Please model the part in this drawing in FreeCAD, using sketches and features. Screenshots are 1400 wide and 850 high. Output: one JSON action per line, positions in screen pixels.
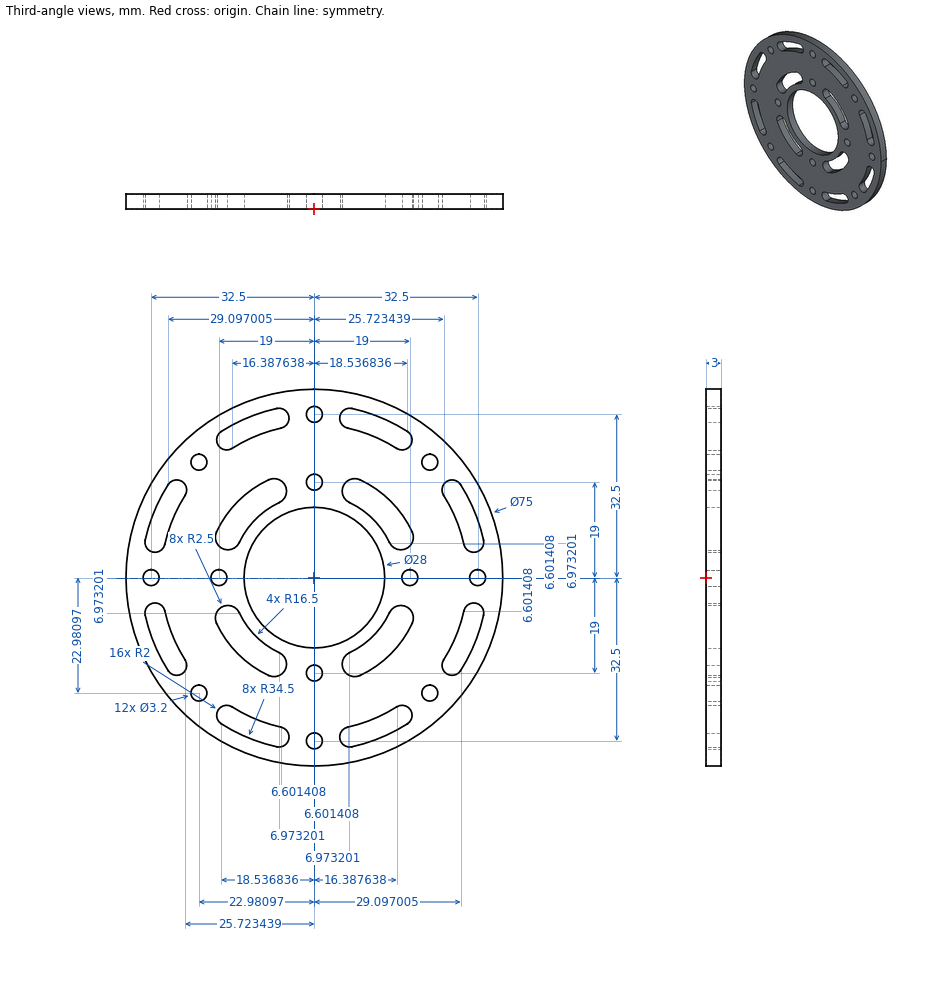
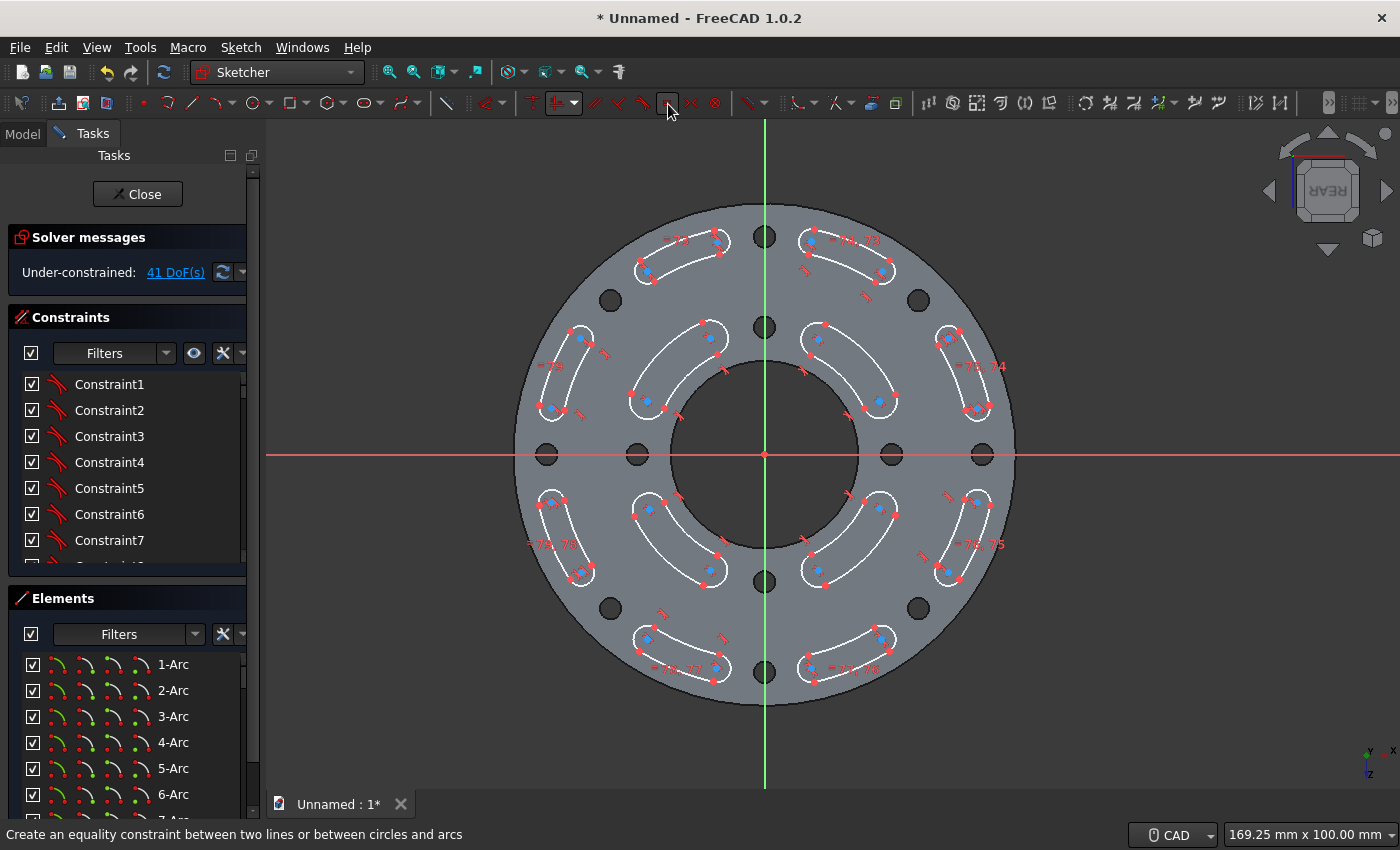
{"action": "scroll", "coordinate": [729, 247], "scroll_direction": "up", "scroll_amount": 2}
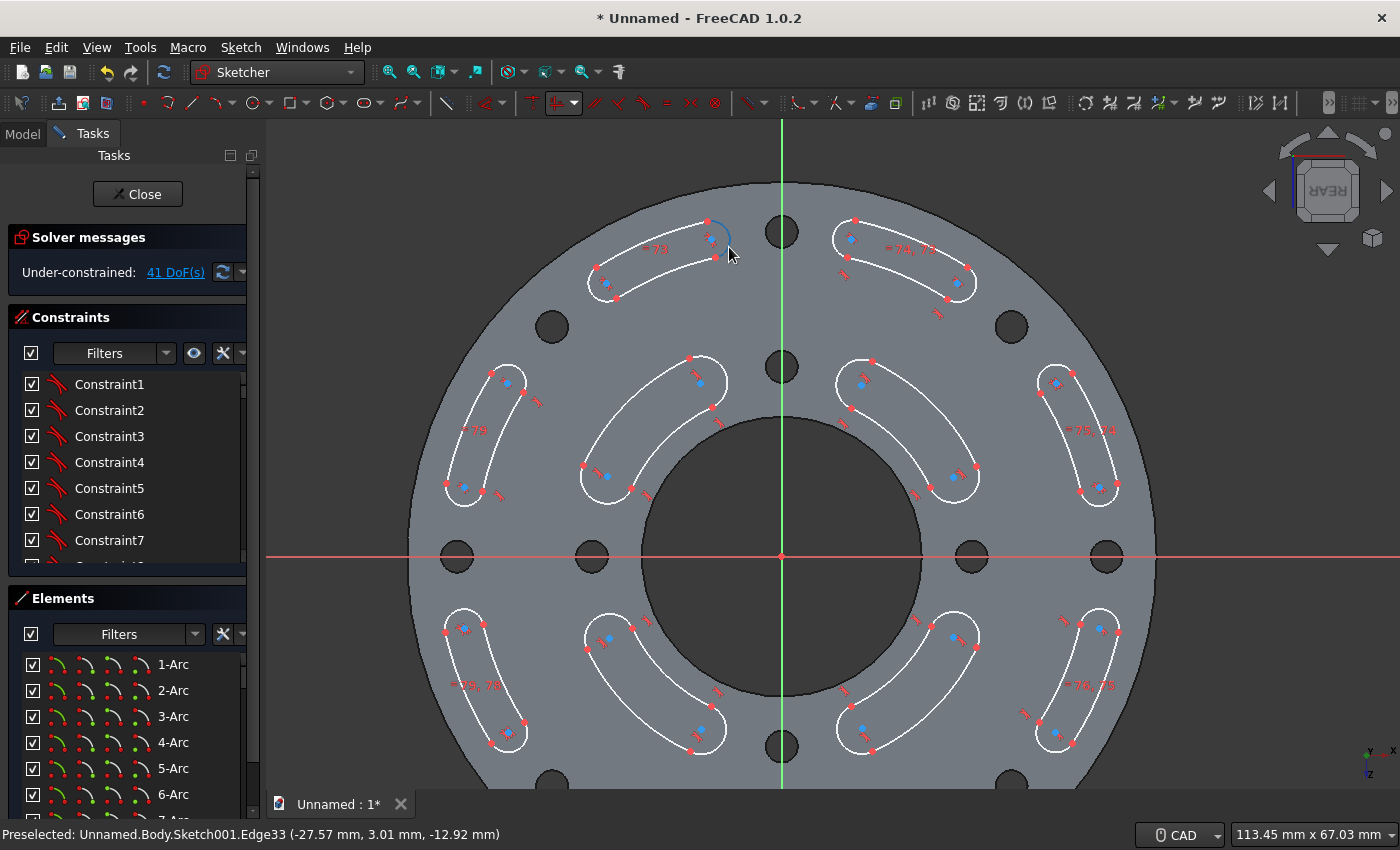
{"action": "left_click", "coordinate": [728, 247]}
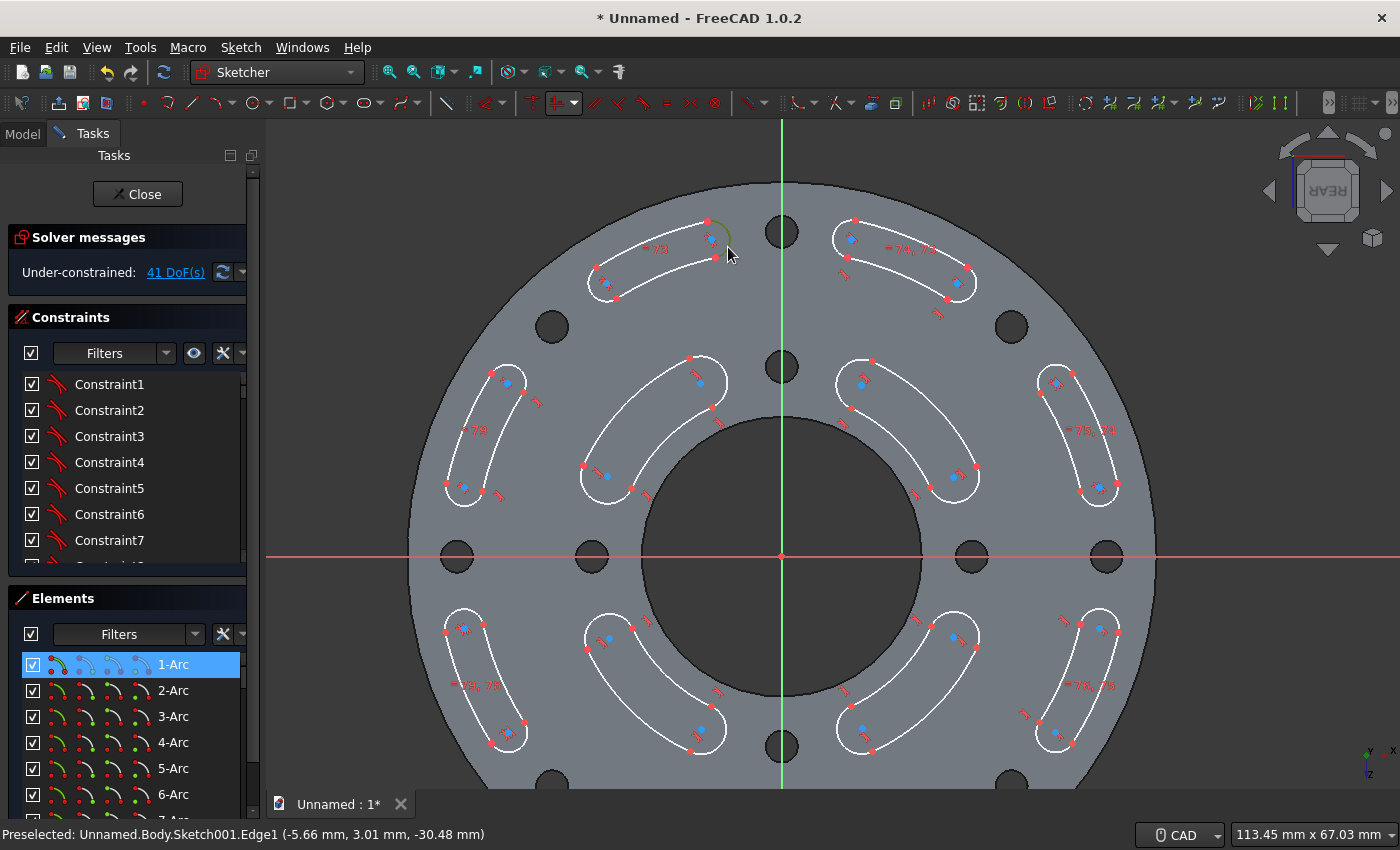
{"action": "left_click", "coordinate": [964, 301]}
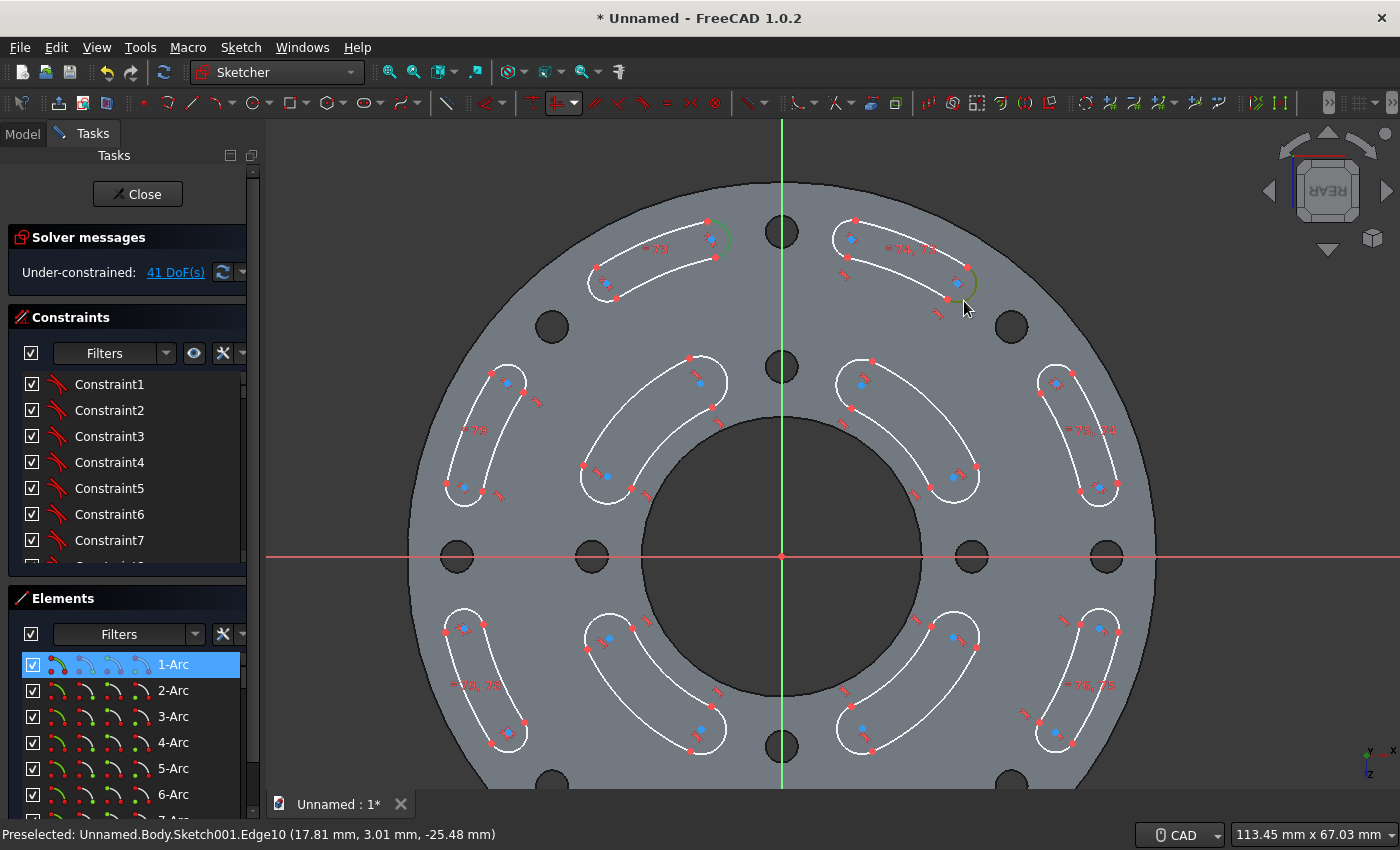
{"action": "left_click", "coordinate": [1092, 505]}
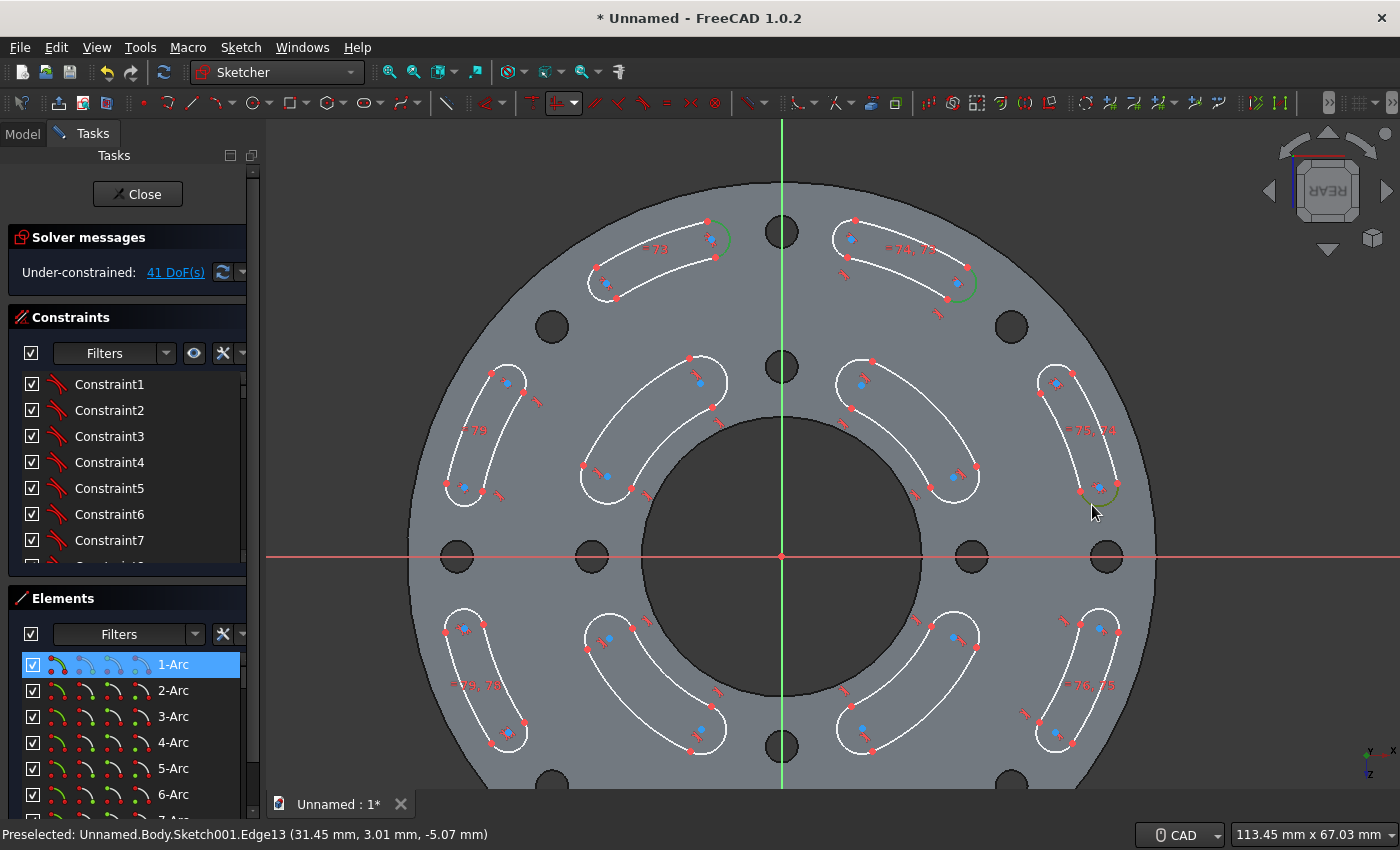
{"action": "left_click", "coordinate": [1038, 740]}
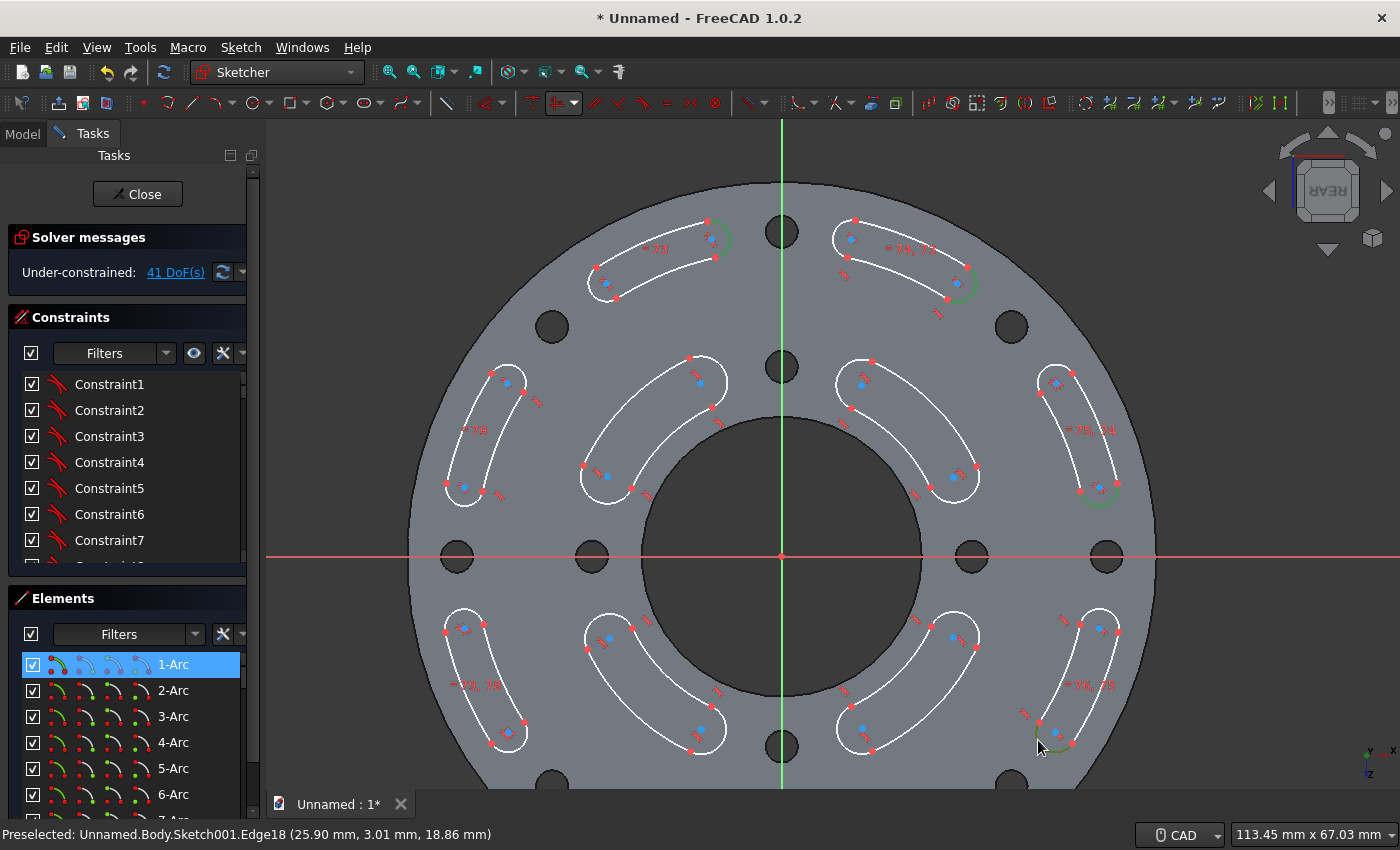
{"action": "scroll", "coordinate": [729, 245], "scroll_direction": "down", "scroll_amount": 2}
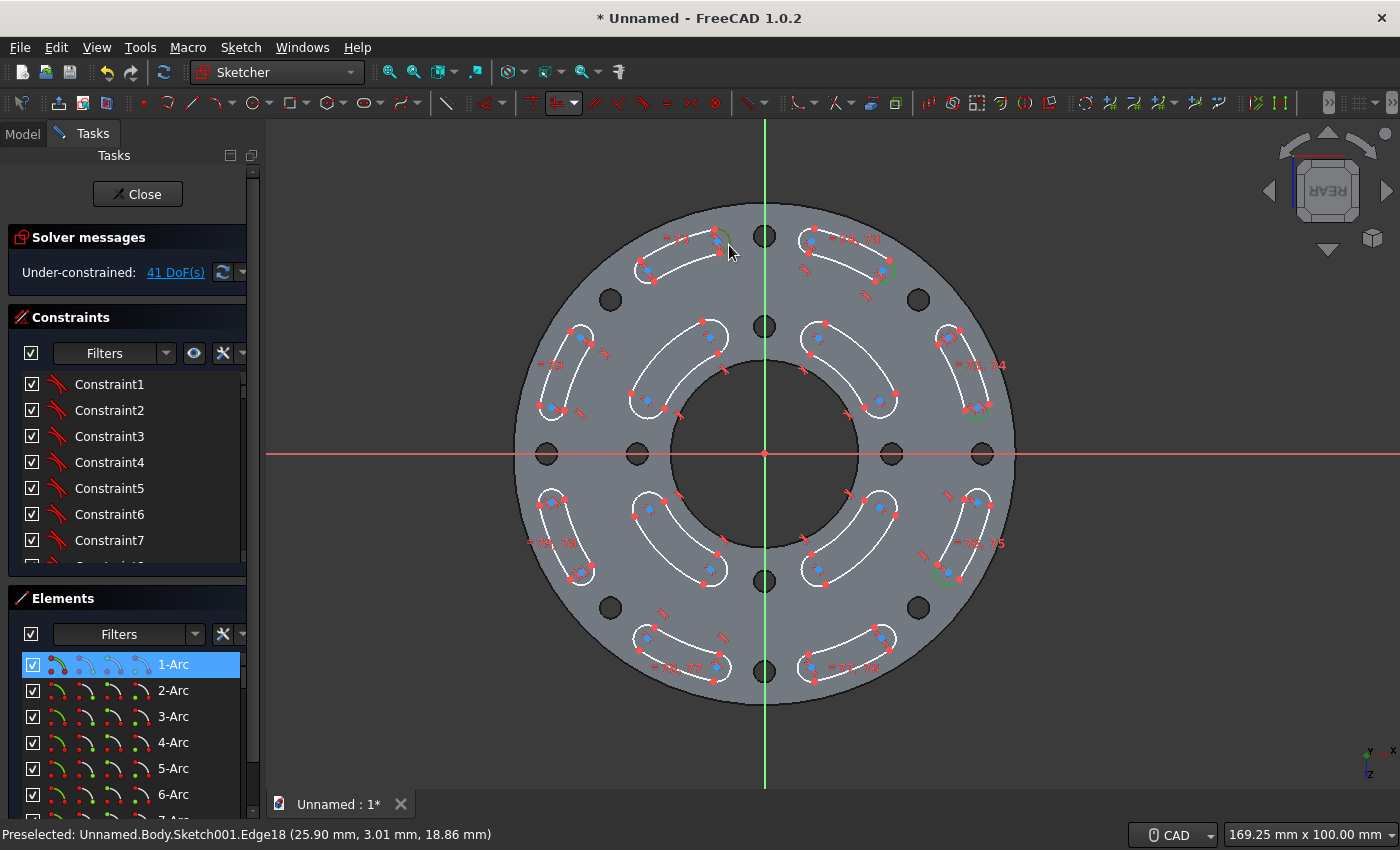
{"action": "left_click", "coordinate": [799, 662]}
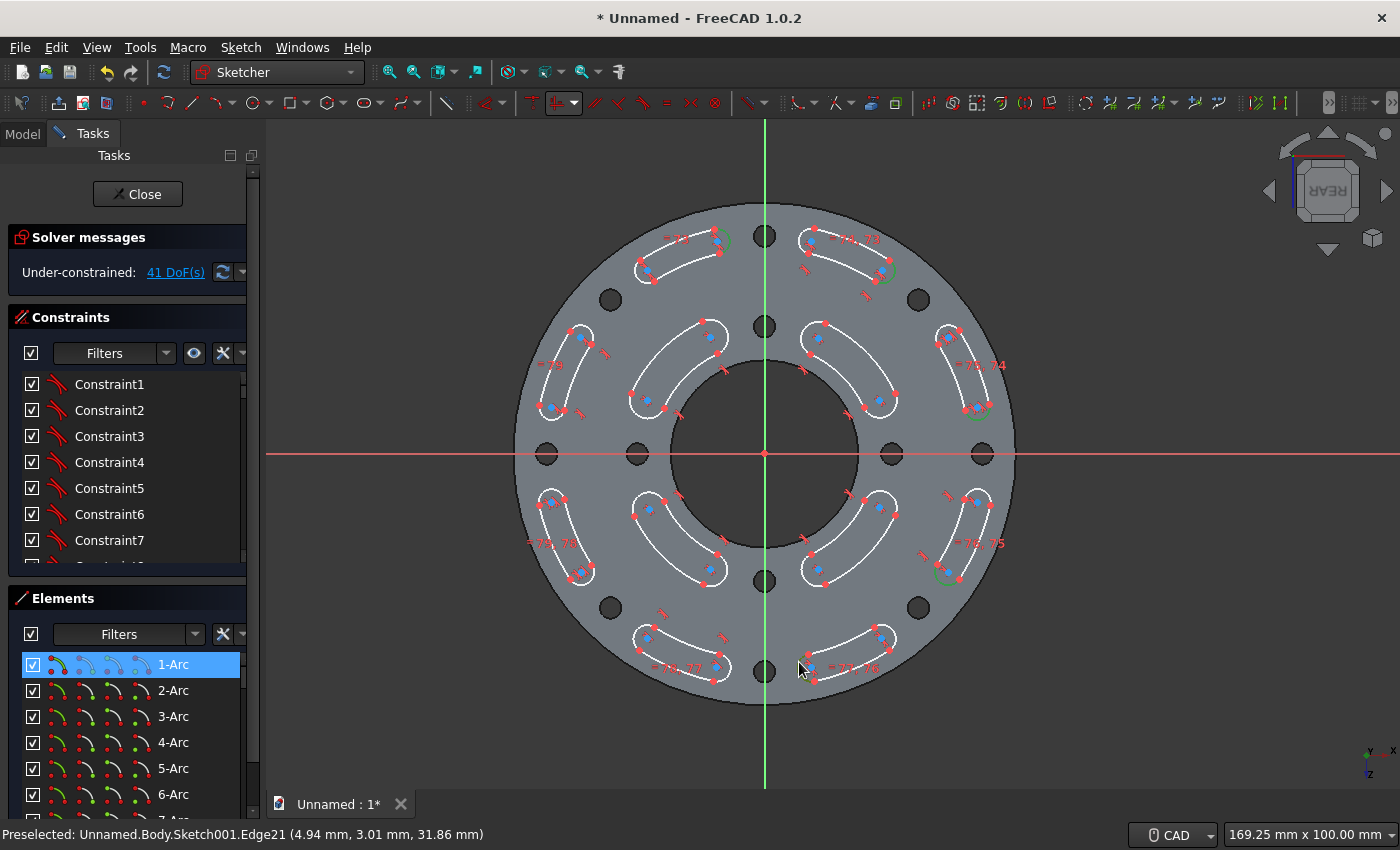
{"action": "left_click", "coordinate": [642, 626]}